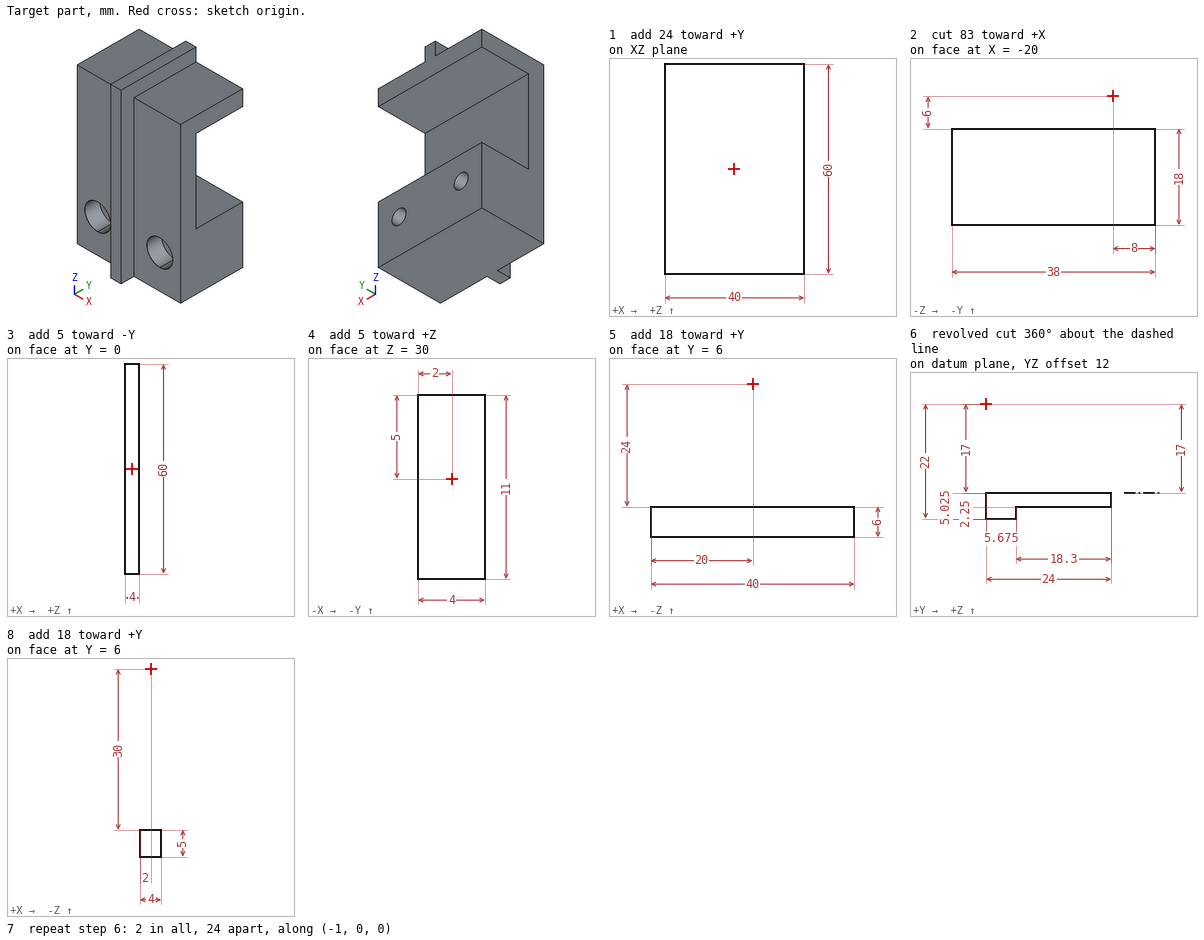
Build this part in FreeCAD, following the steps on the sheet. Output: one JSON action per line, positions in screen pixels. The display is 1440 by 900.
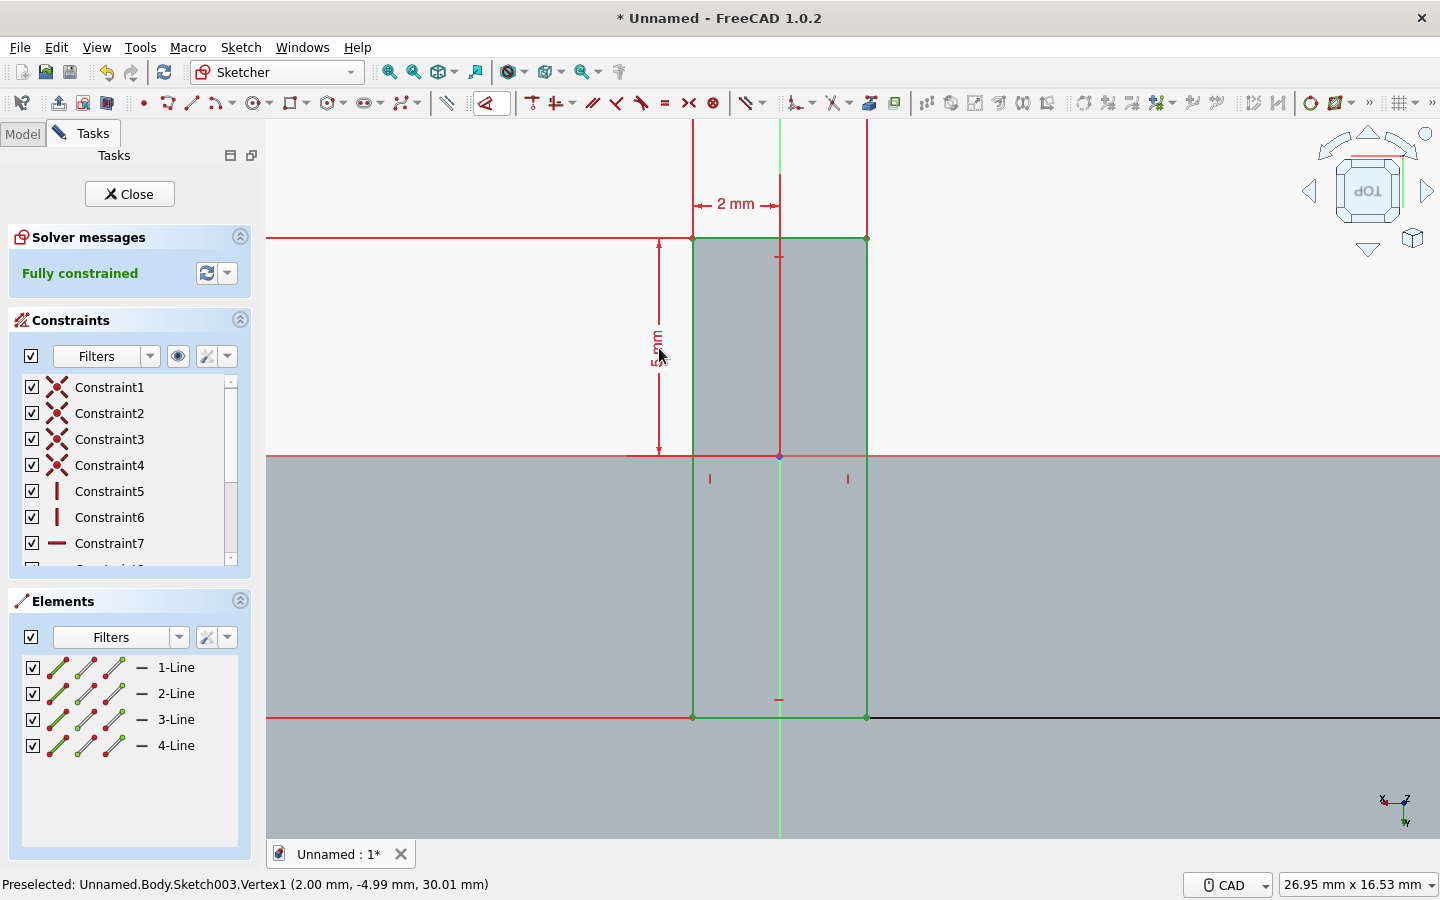
{"action": "left_click", "coordinate": [130, 194]}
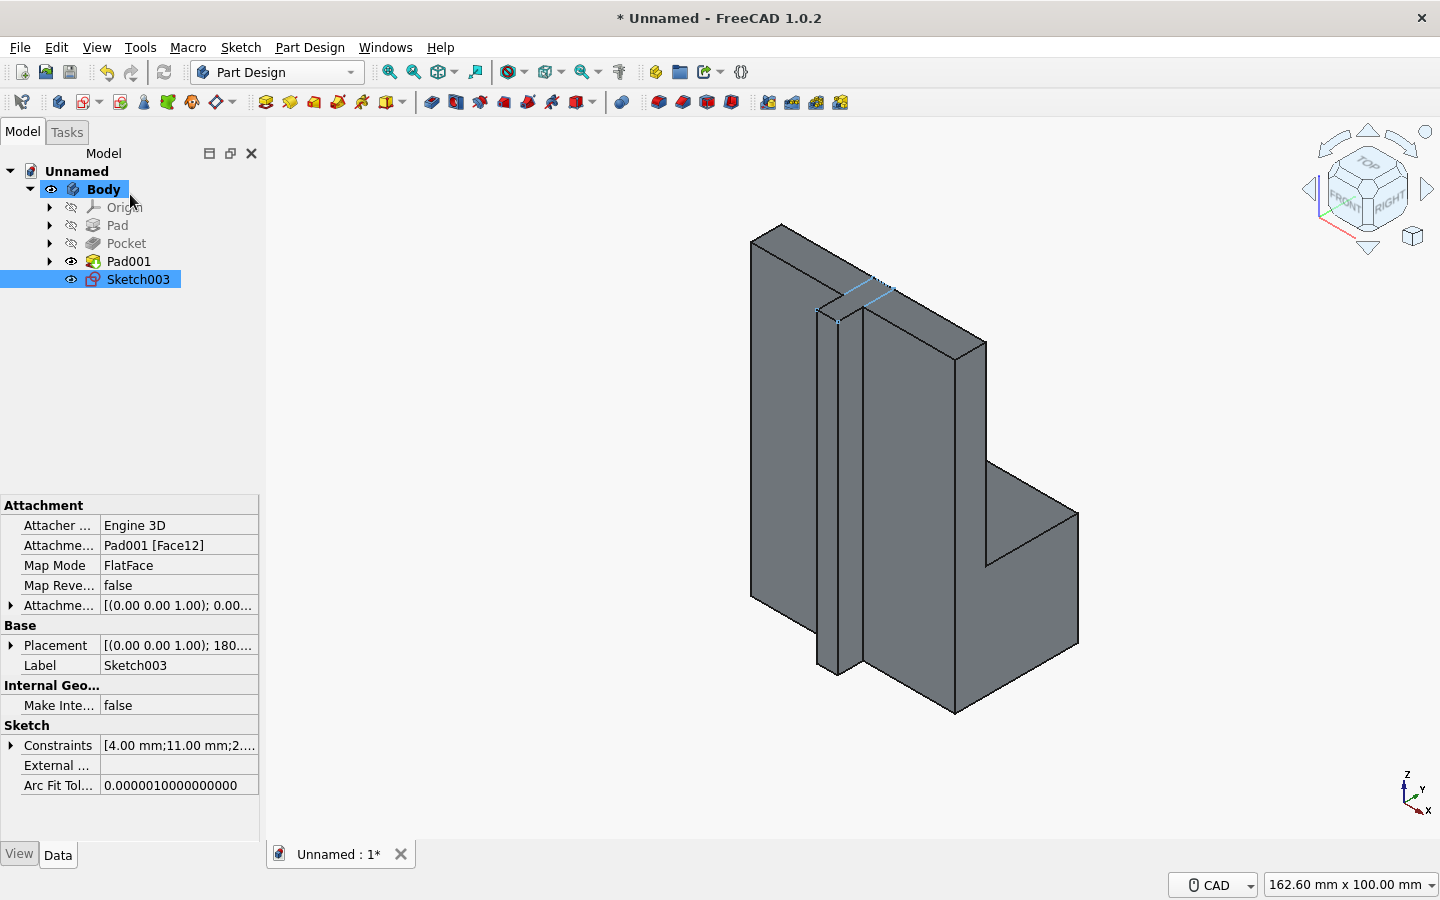
{"action": "left_click", "coordinate": [266, 102]}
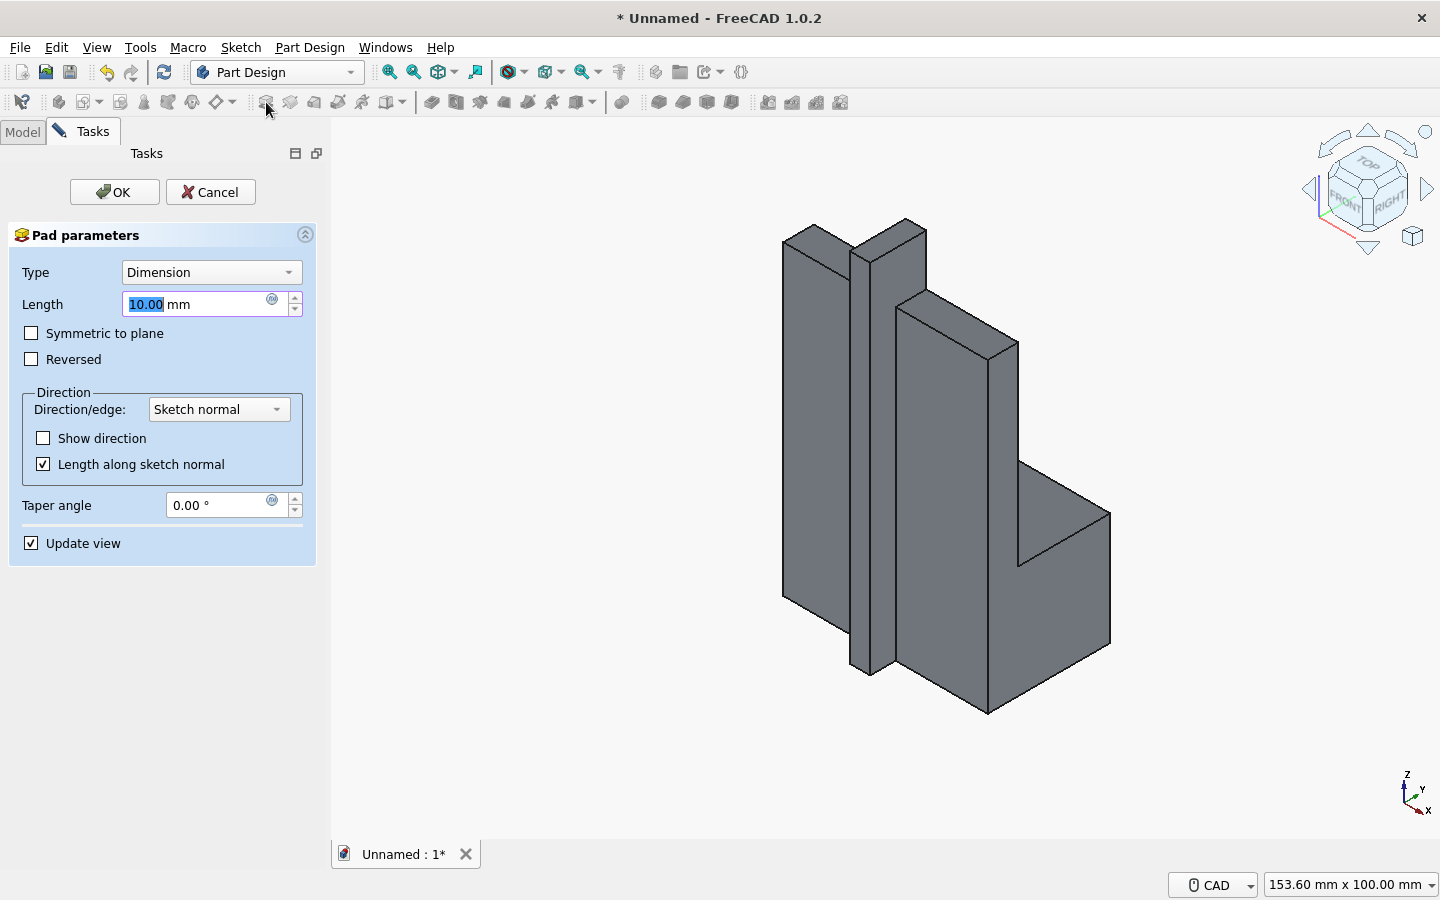
{"action": "type", "text": "5"}
{"action": "key", "text": "Tab"}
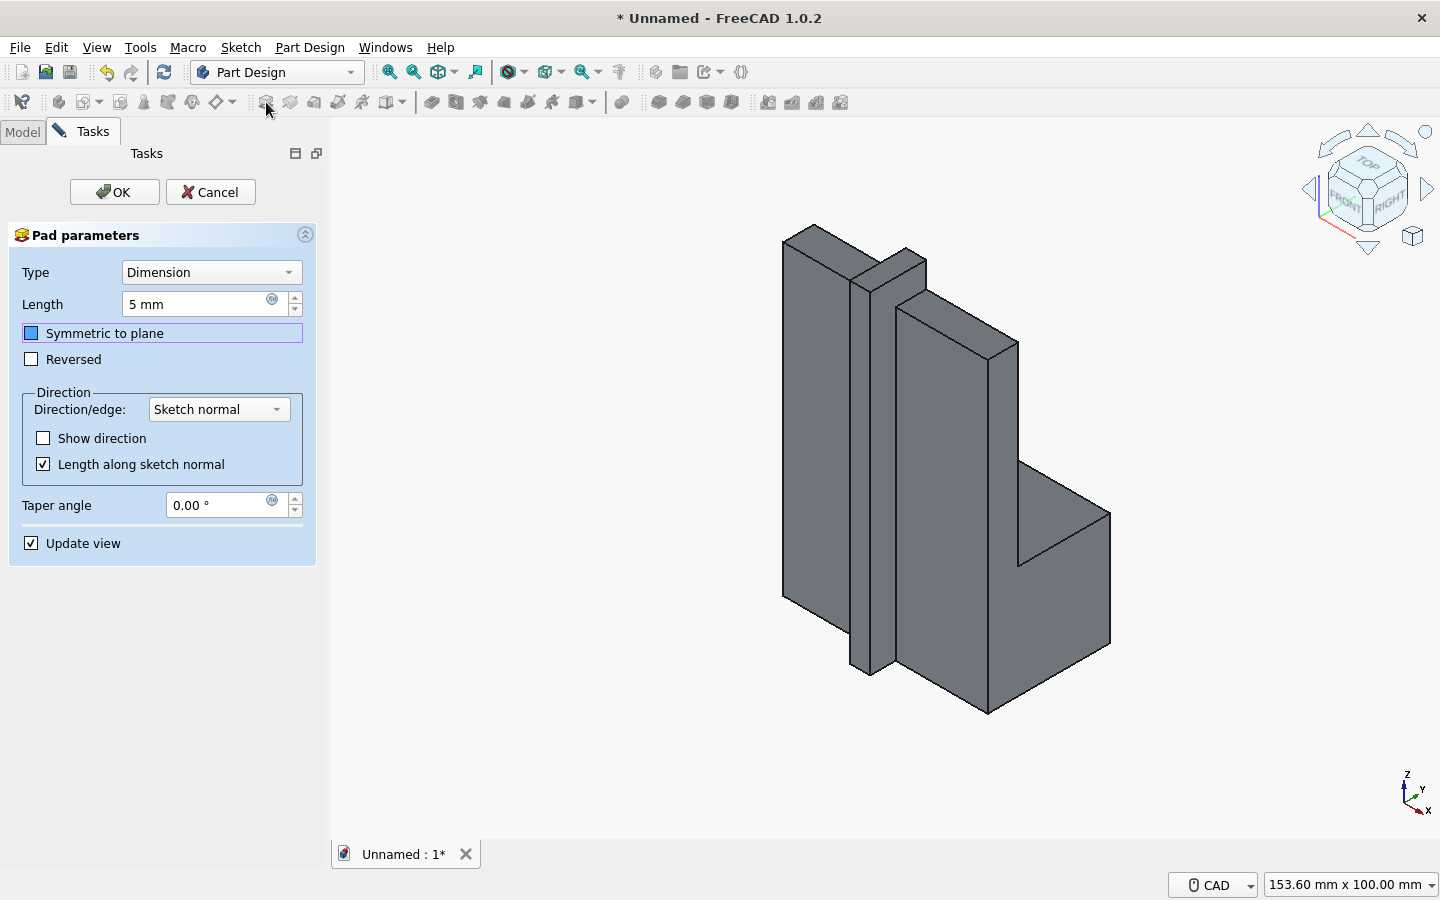
{"action": "left_click", "coordinate": [115, 192]}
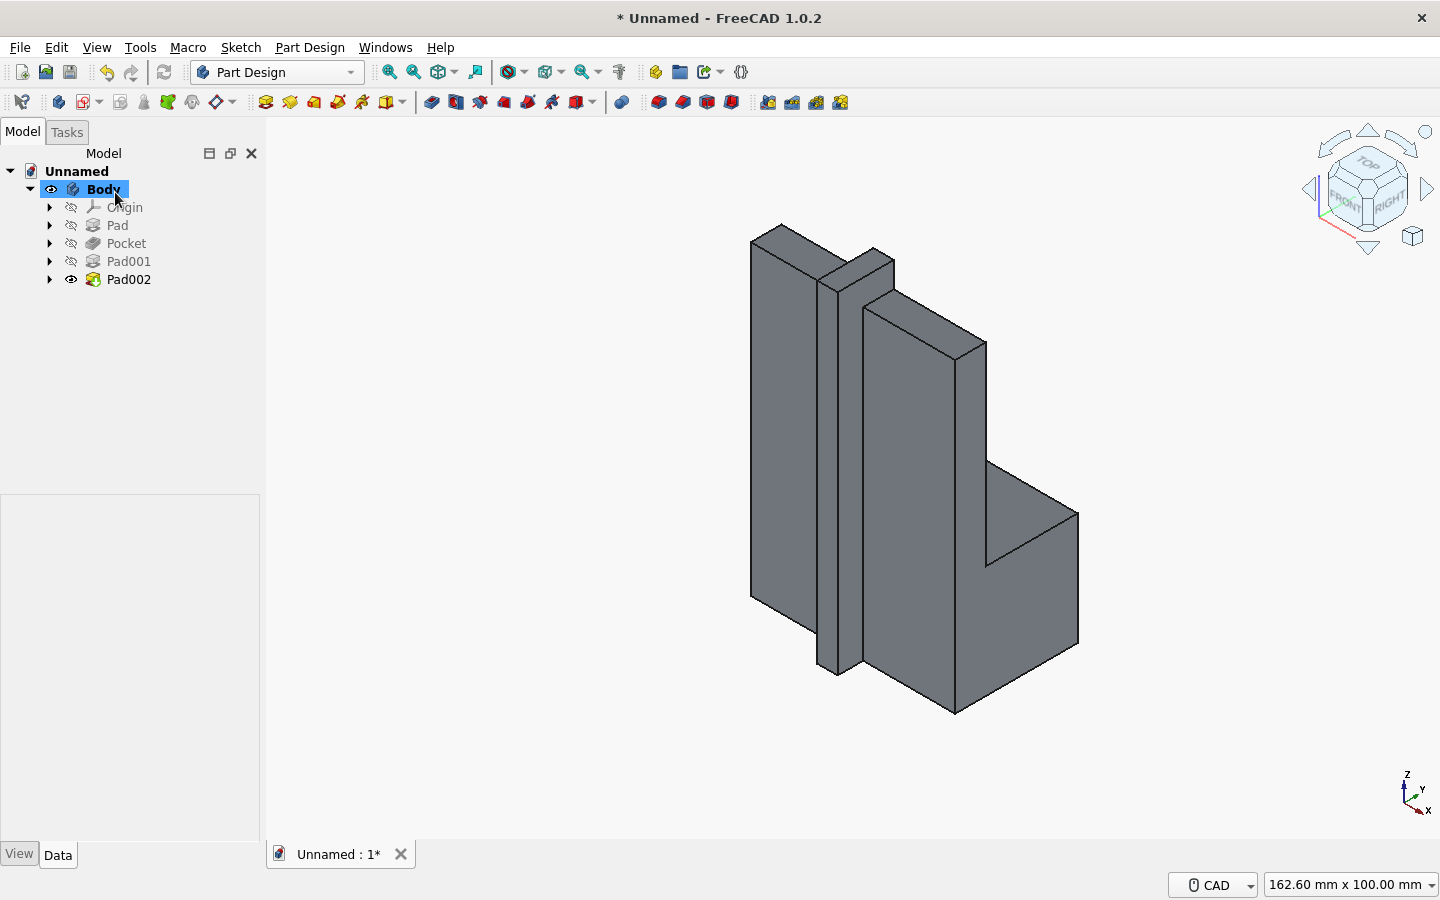
{"action": "key", "text": "4"}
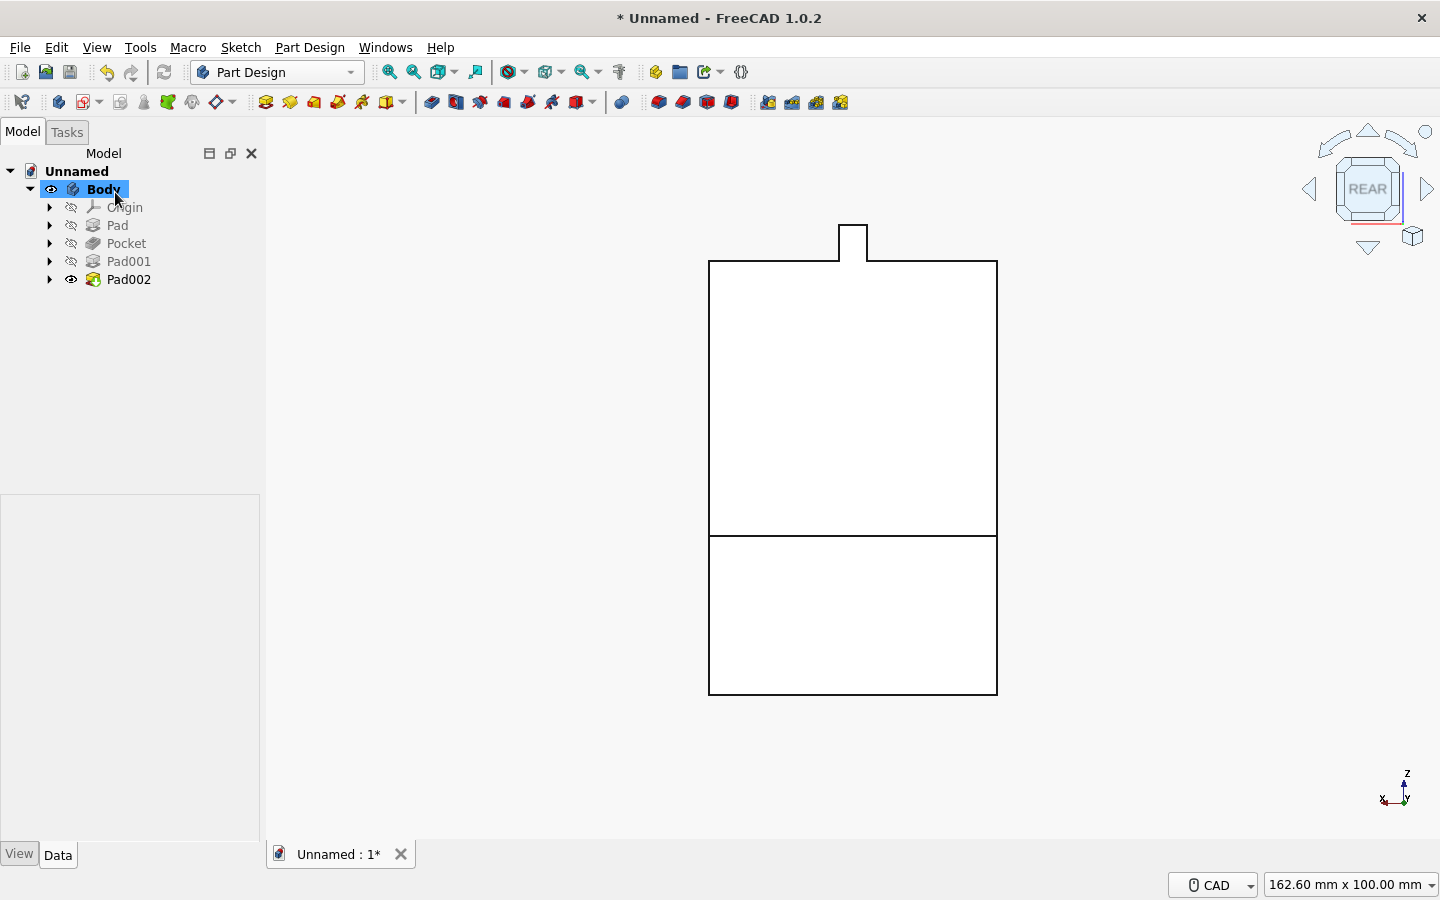
{"action": "left_click", "coordinate": [853, 380]}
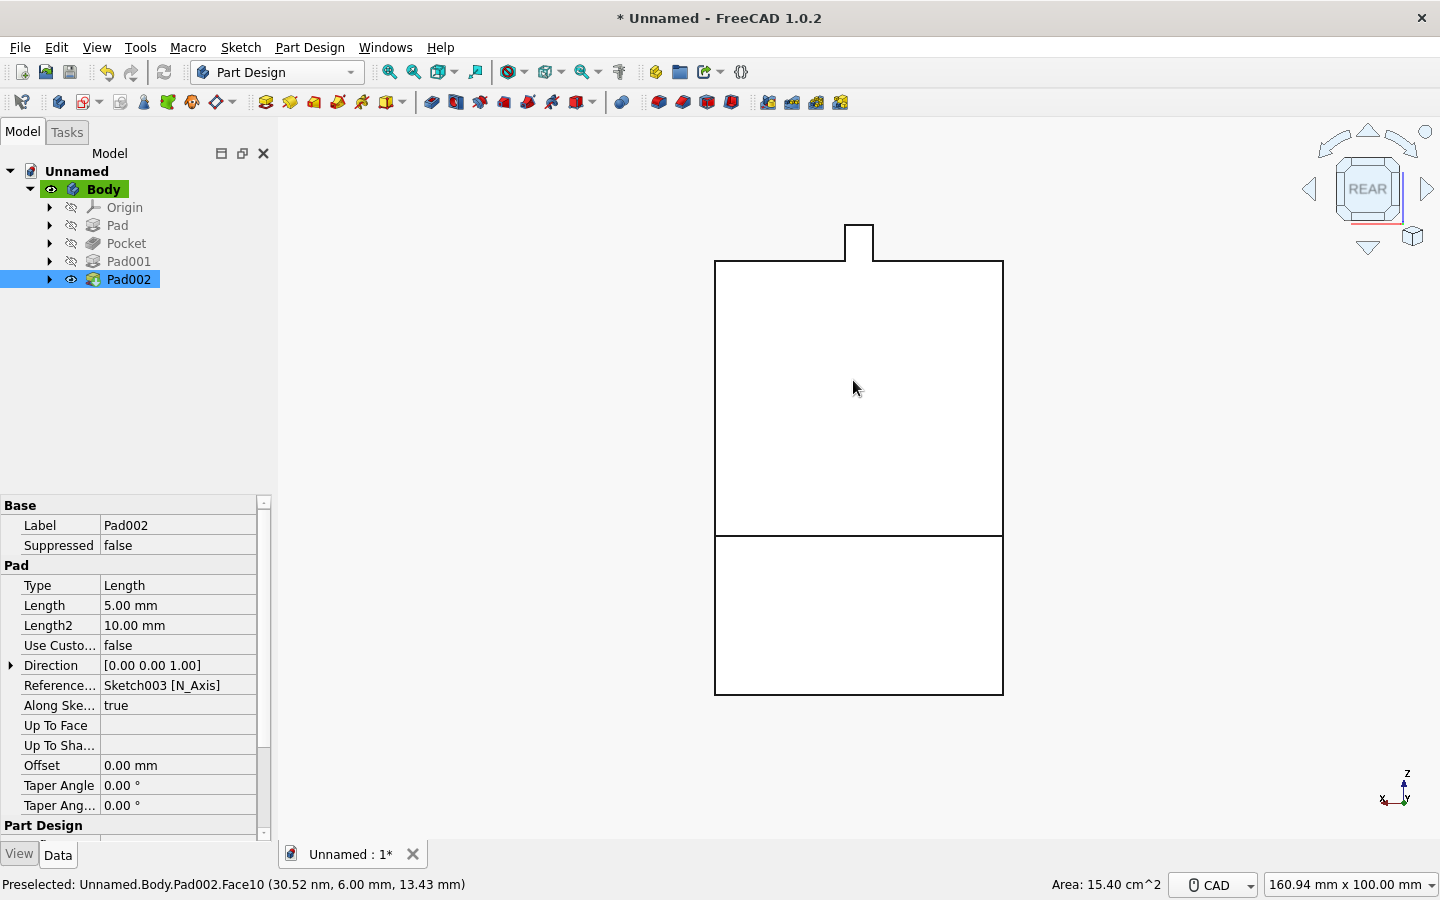
{"action": "left_click", "coordinate": [84, 102]}